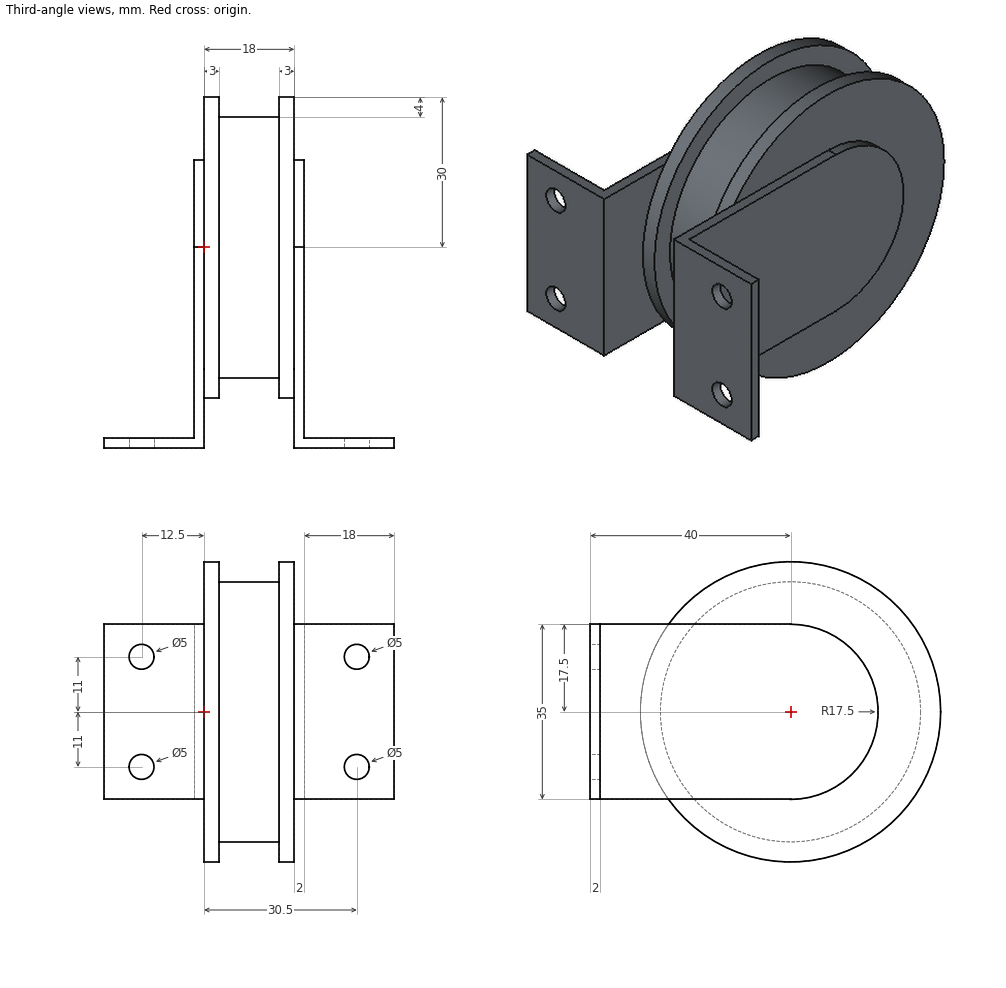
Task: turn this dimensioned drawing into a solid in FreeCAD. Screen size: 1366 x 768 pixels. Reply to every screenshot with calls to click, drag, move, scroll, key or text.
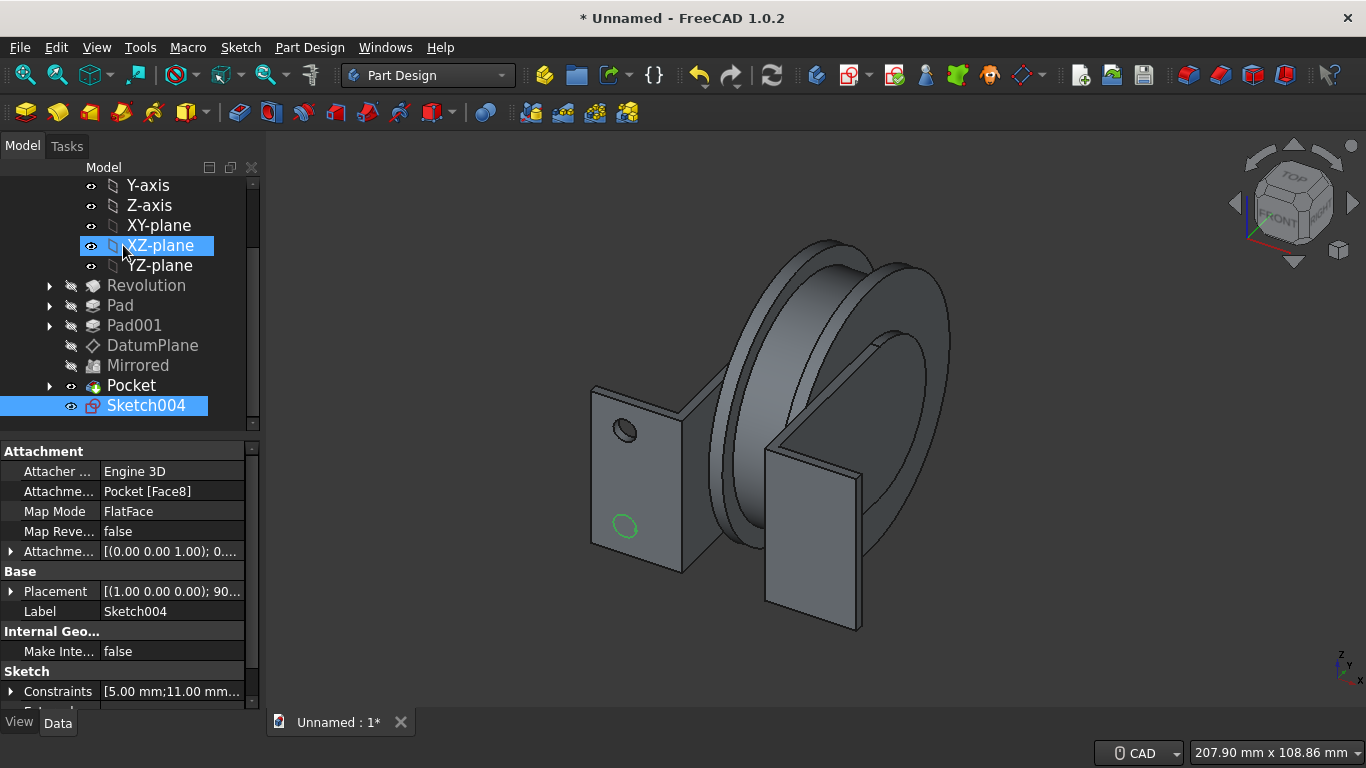
click(240, 112)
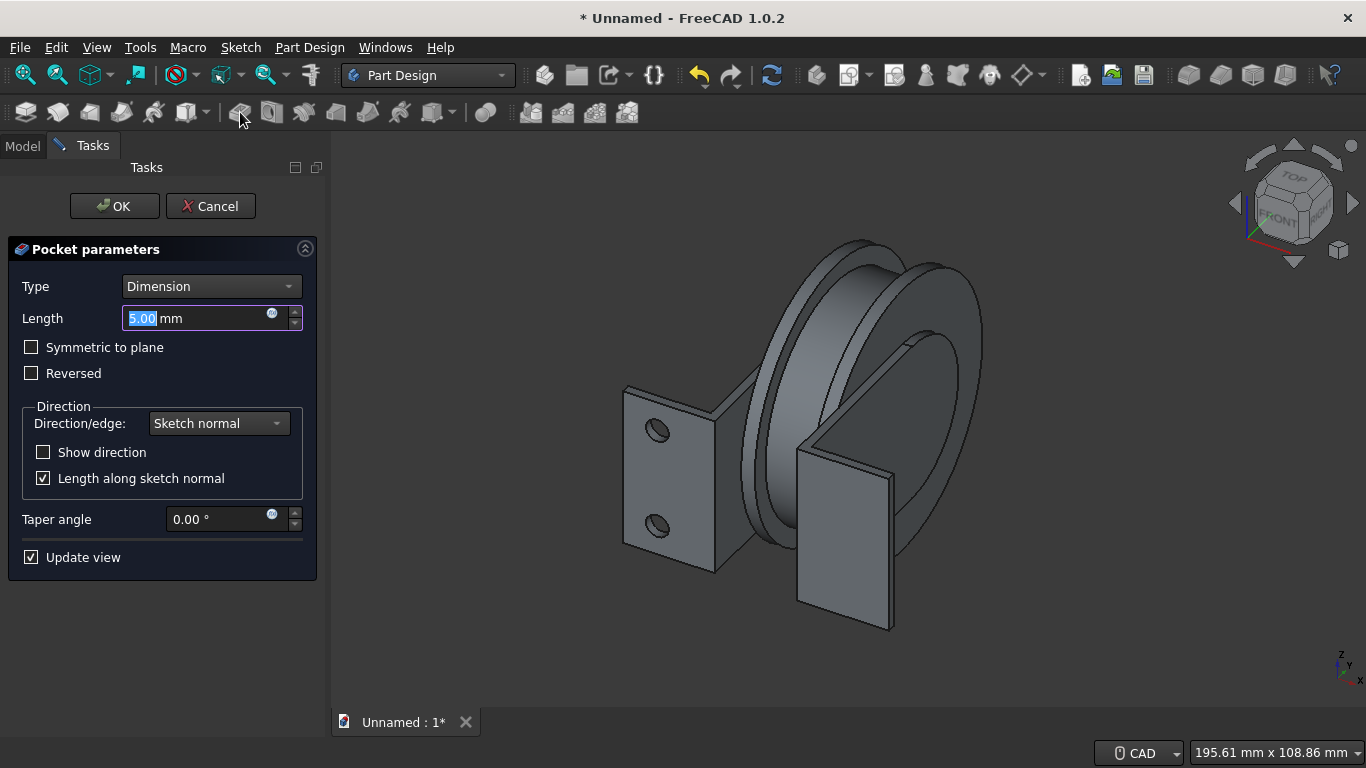
click(212, 286)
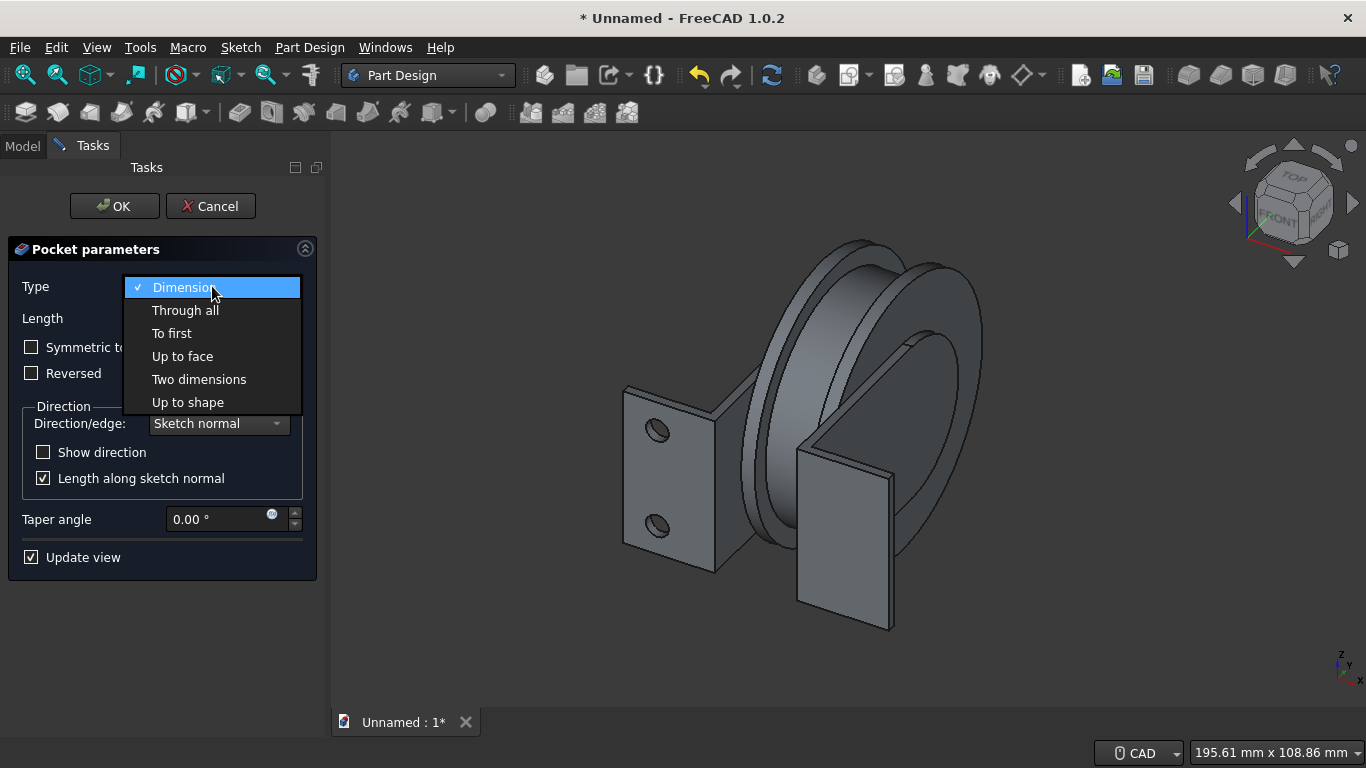
click(212, 334)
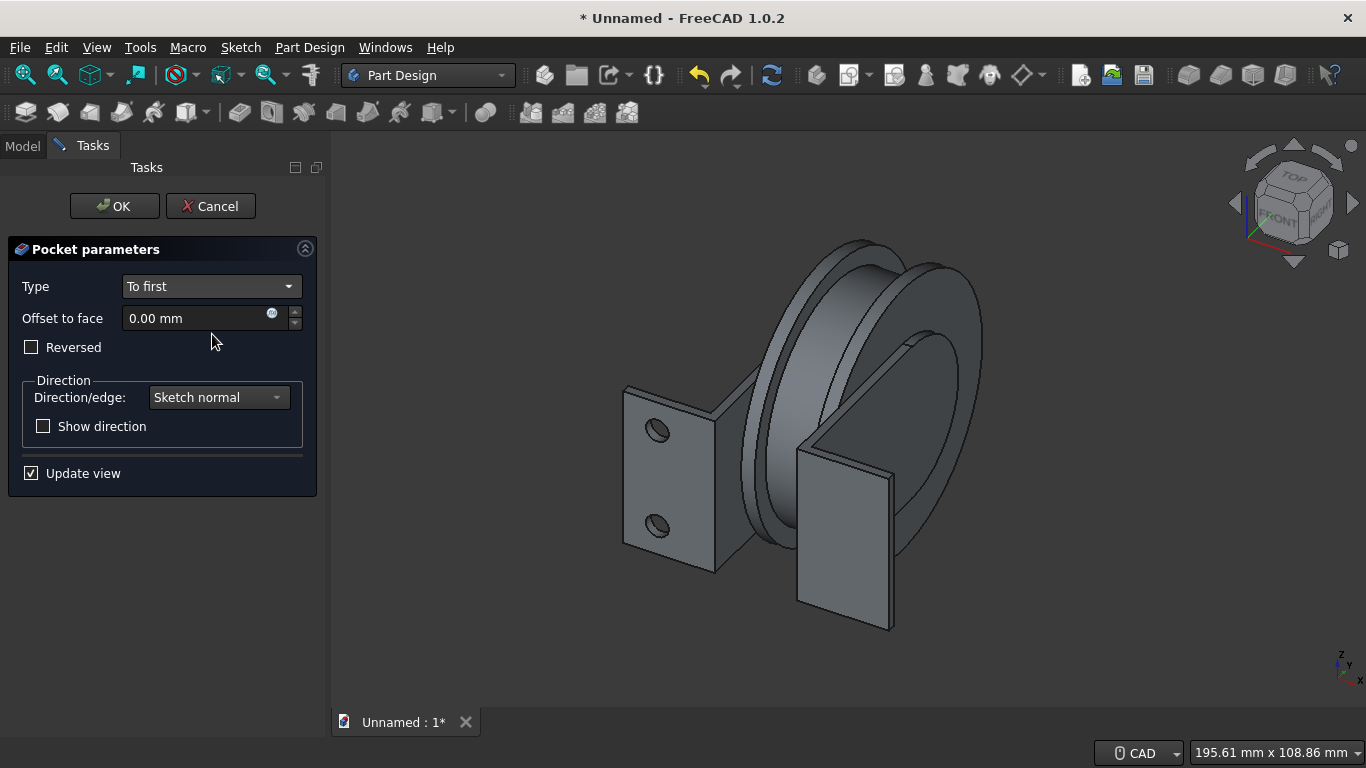
click(115, 206)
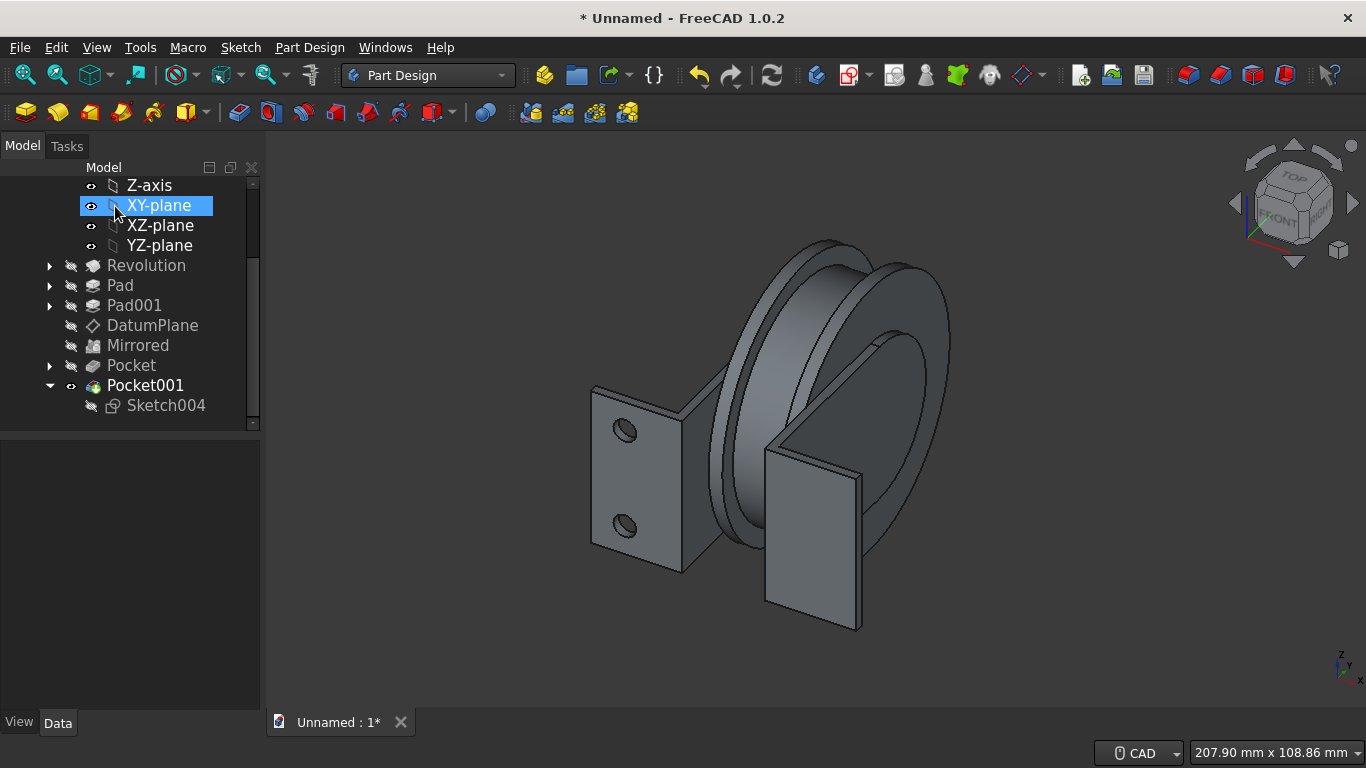
click(810, 517)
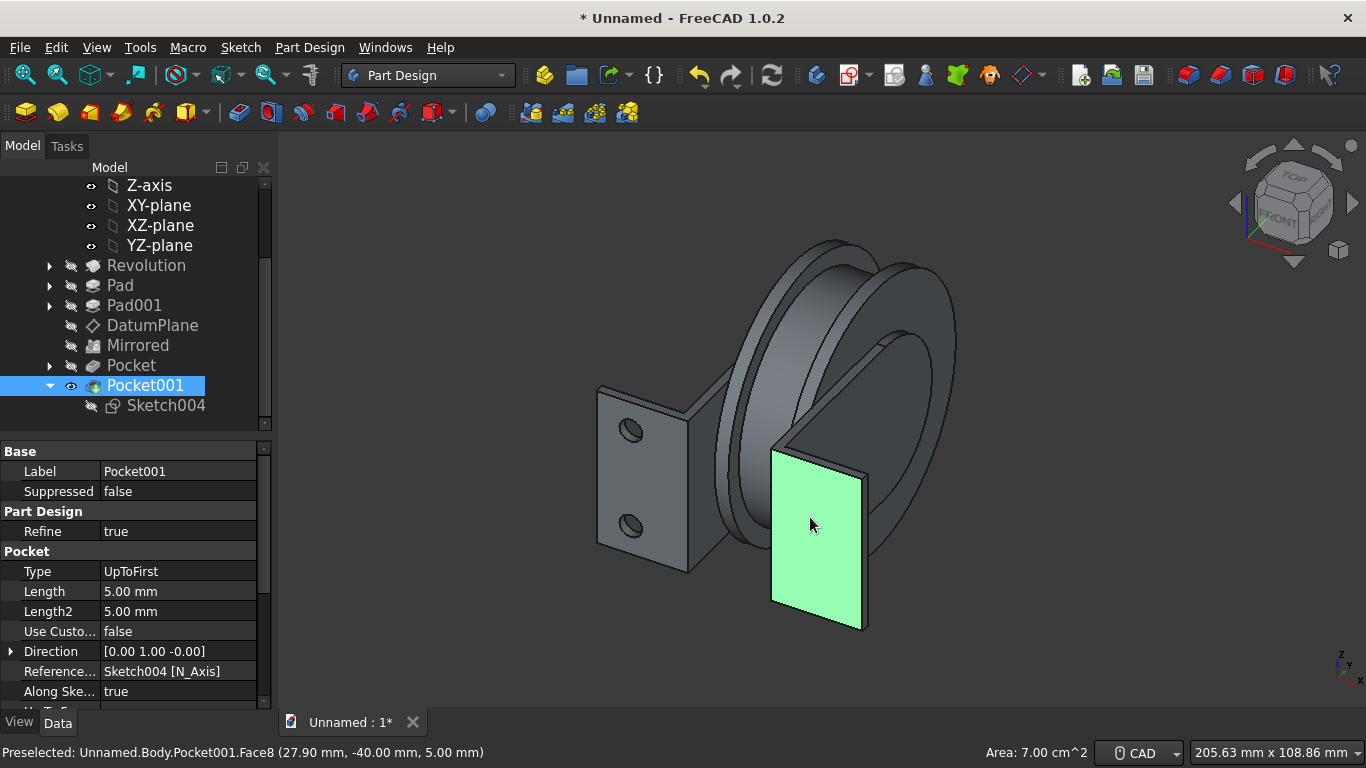
click(850, 76)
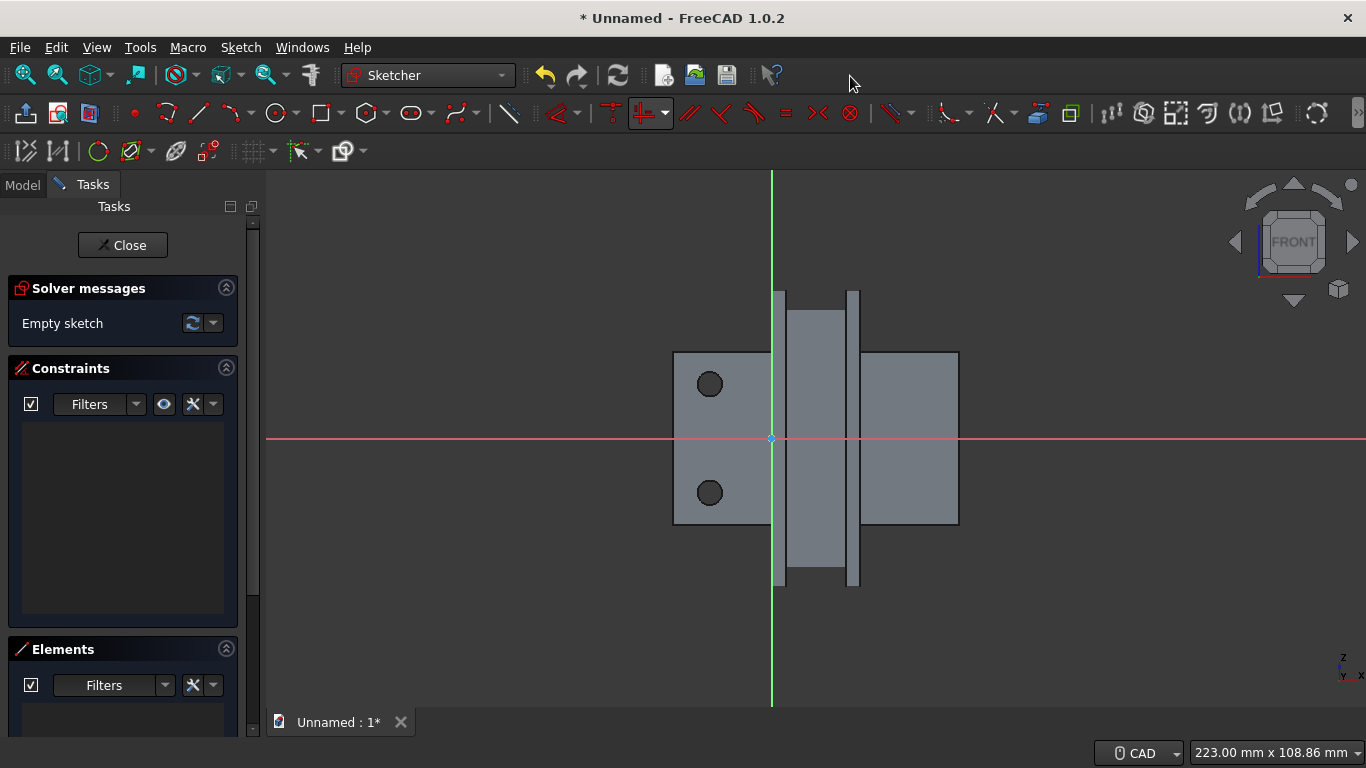
scroll(936, 497, up, 13)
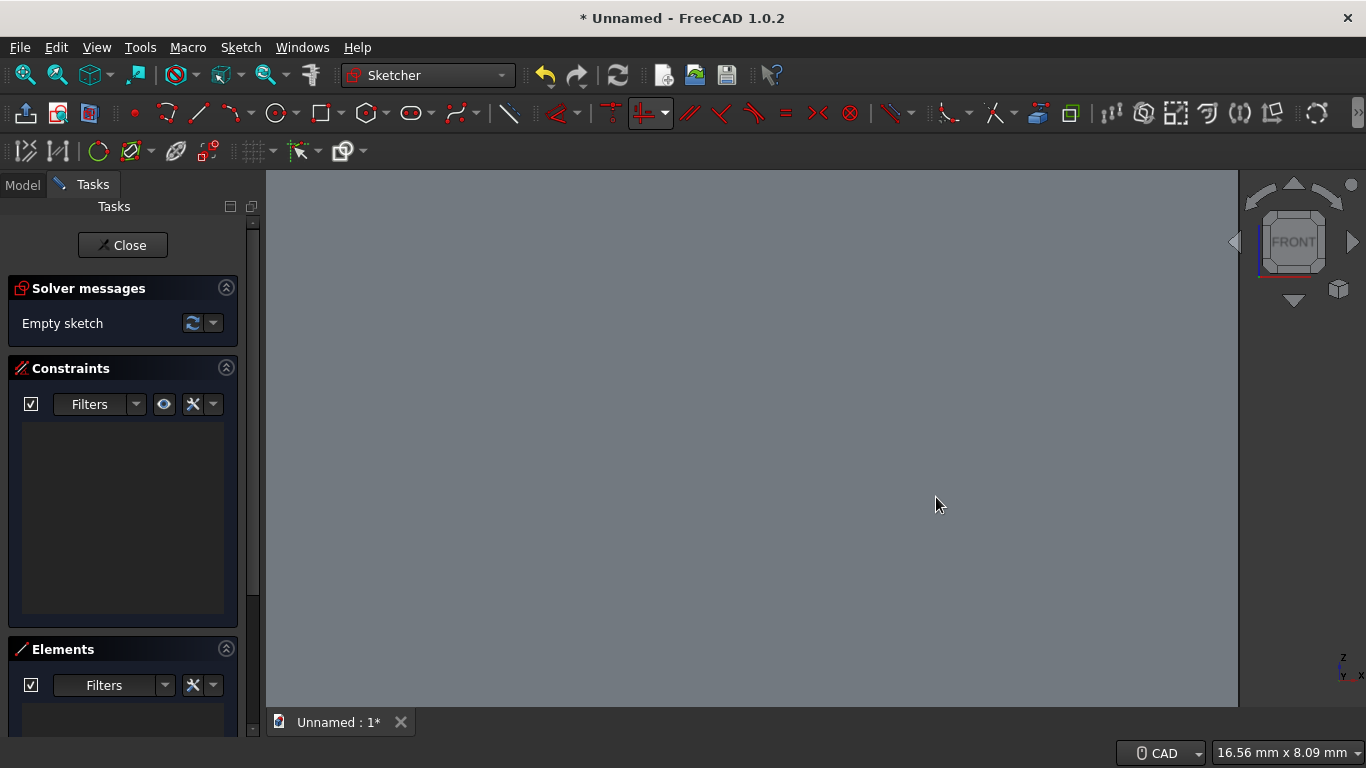
click(276, 114)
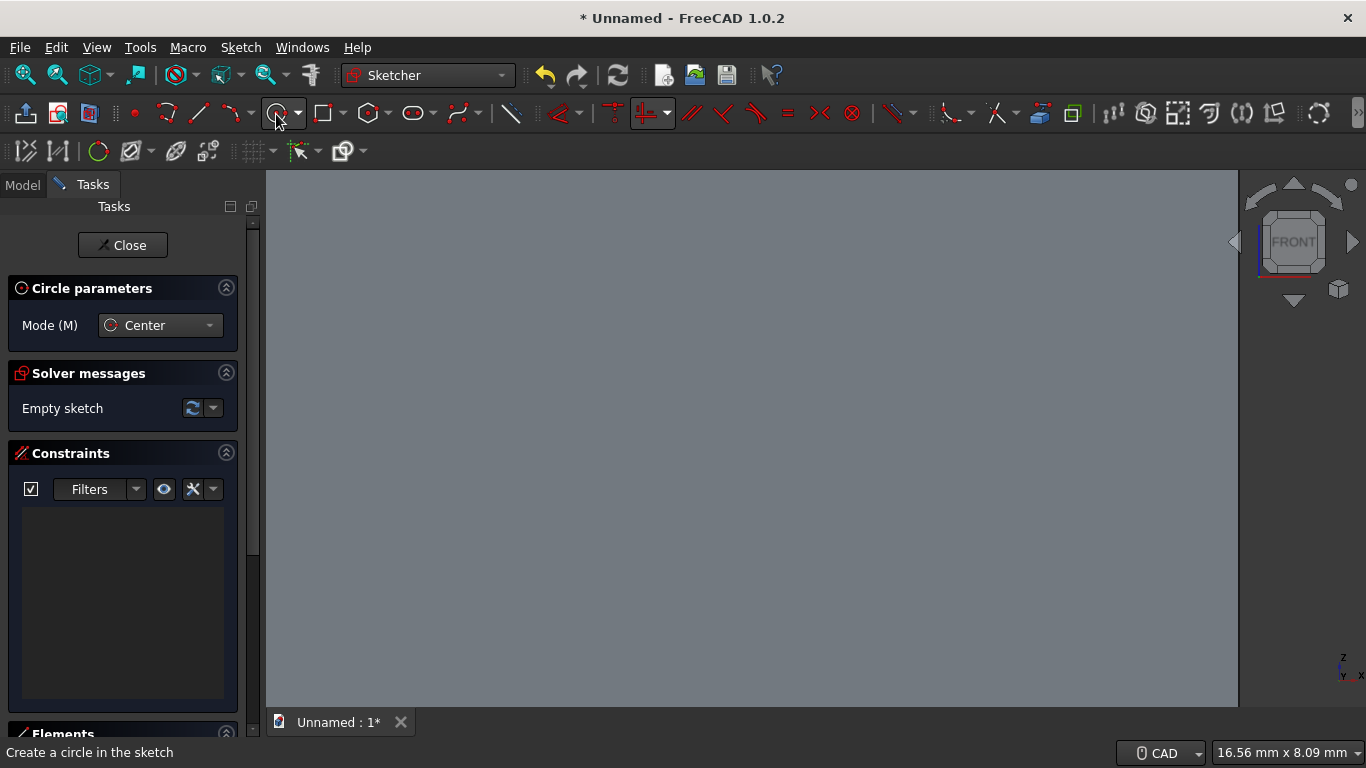
click(741, 432)
click(858, 315)
key(Escape)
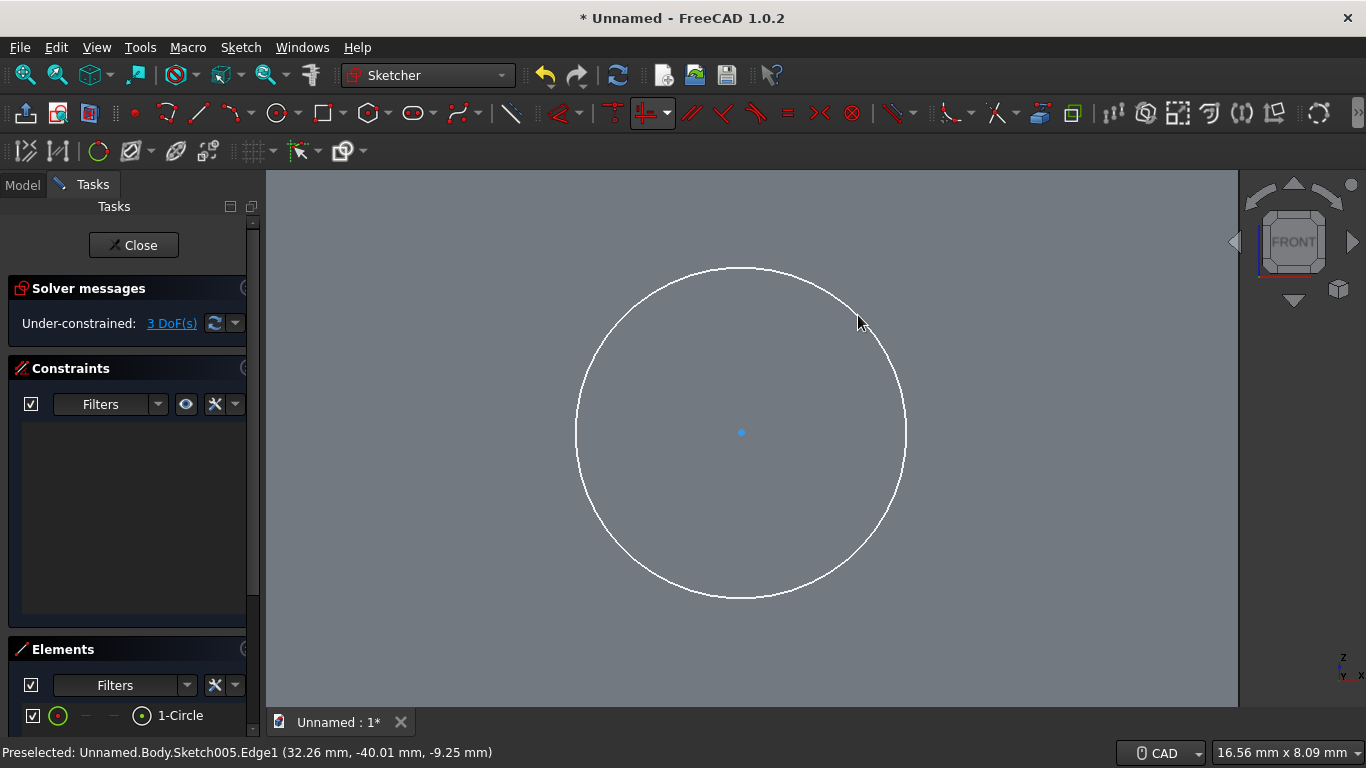
key(d)